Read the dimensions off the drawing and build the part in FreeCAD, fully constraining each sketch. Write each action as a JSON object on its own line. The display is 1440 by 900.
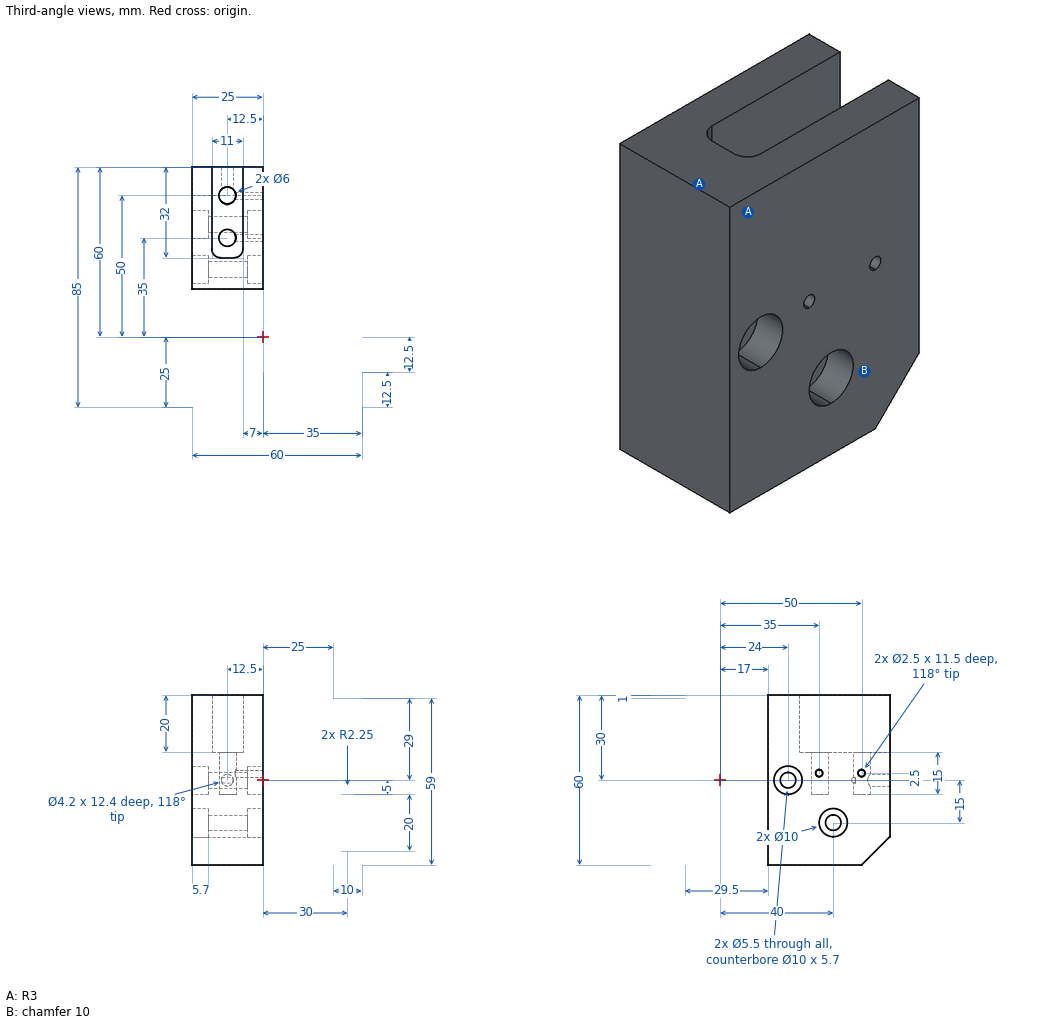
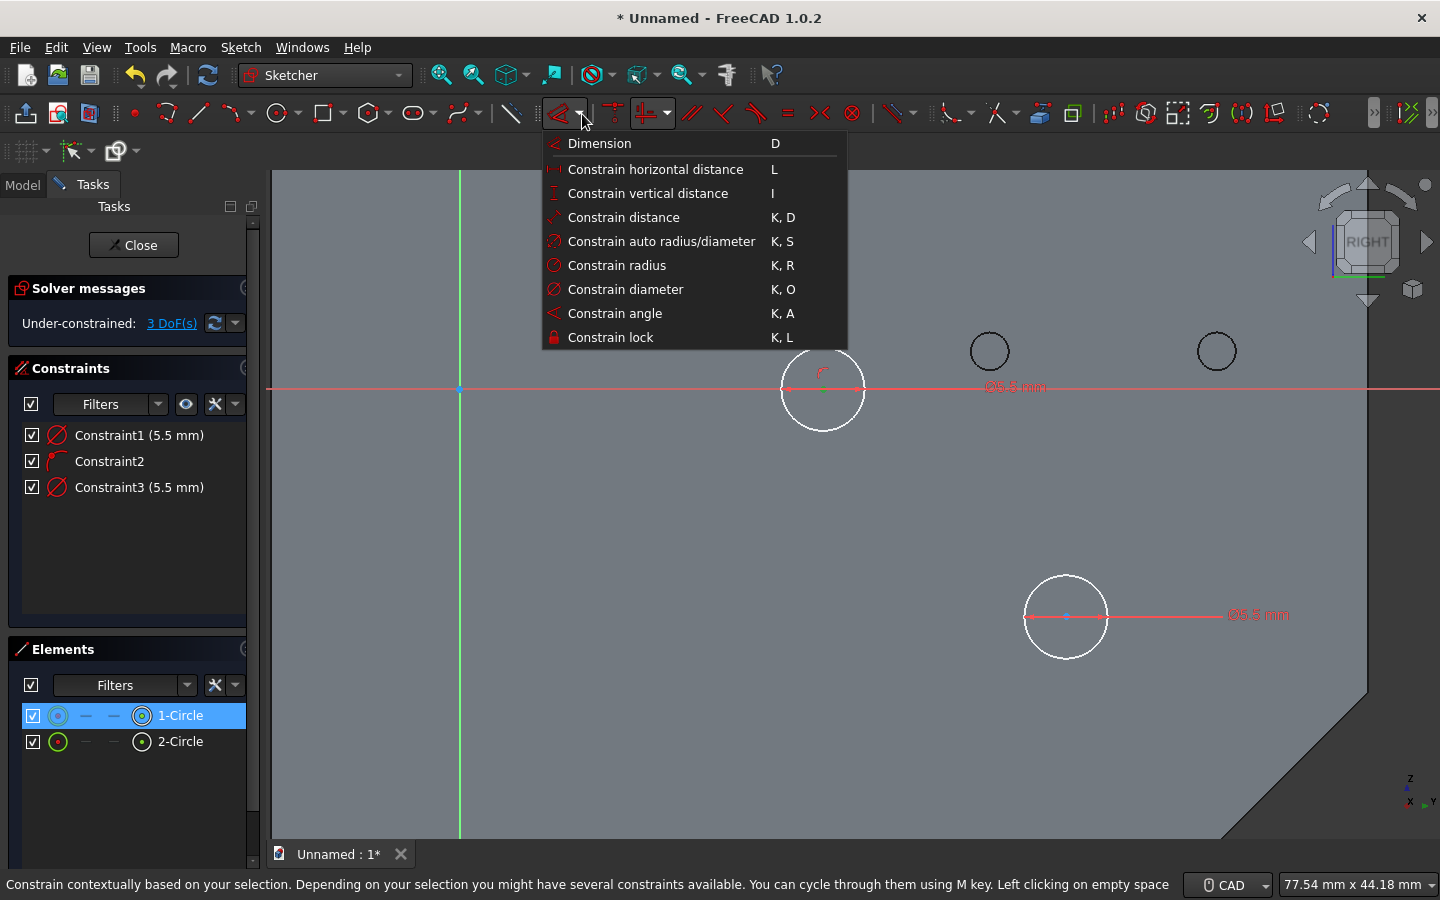
{"action": "left_click", "coordinate": [695, 169]}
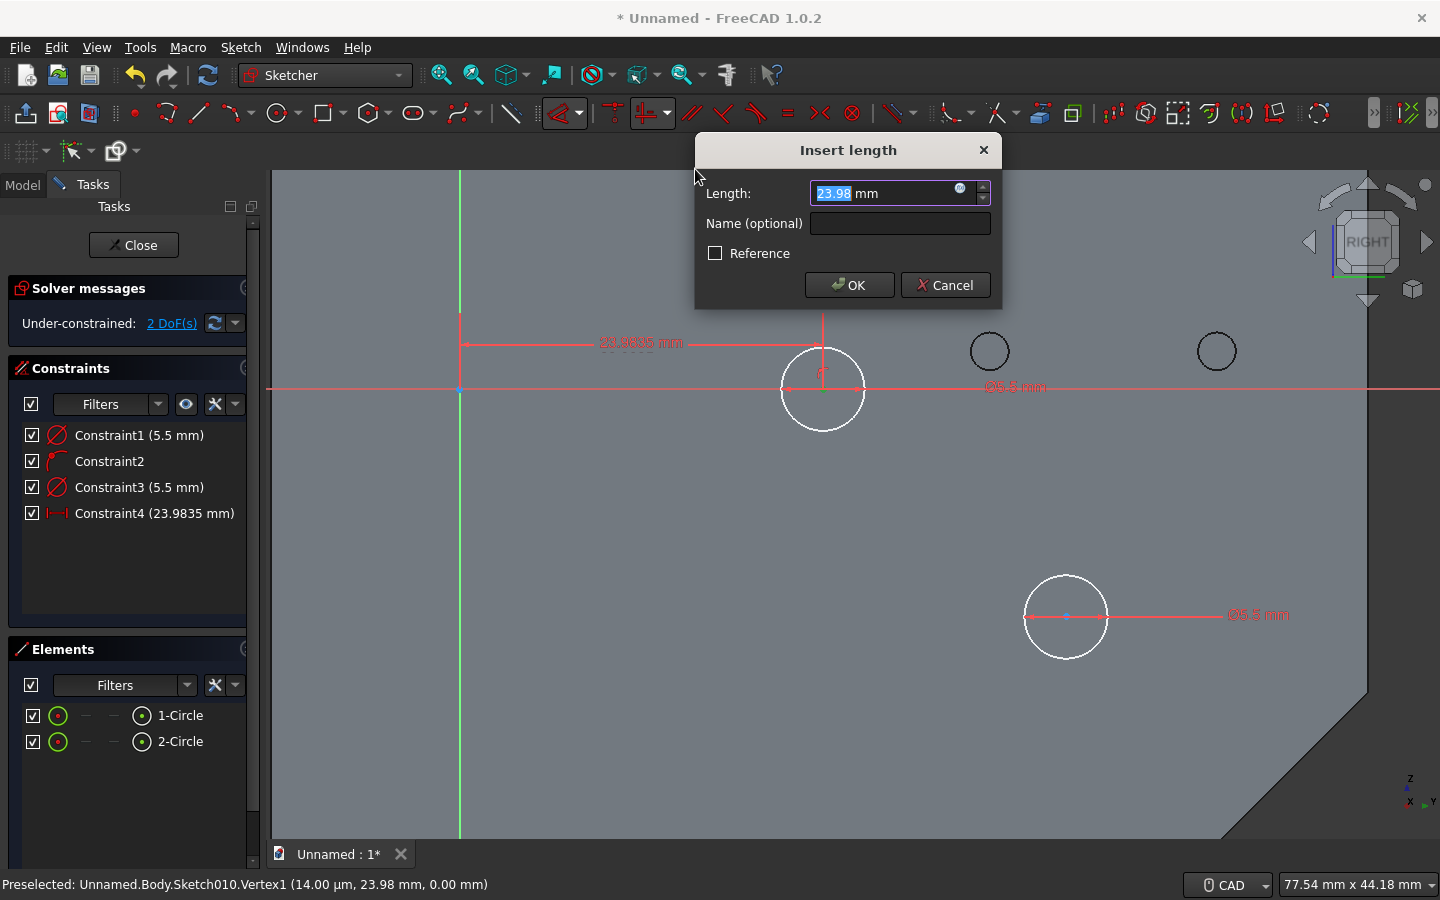
{"action": "type", "text": "24"}
{"action": "key", "text": "Return"}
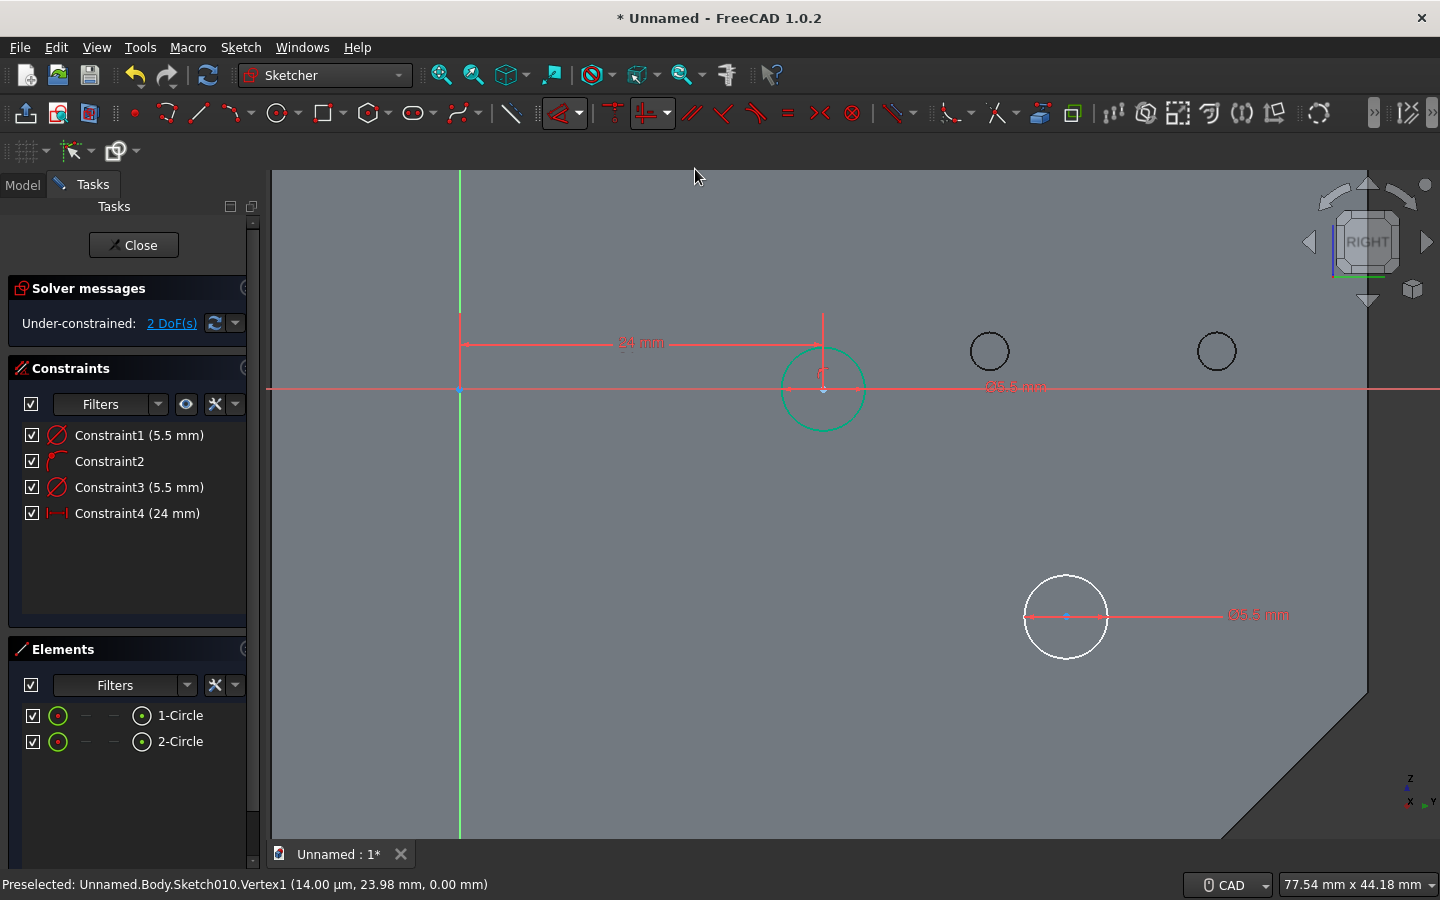
{"action": "left_click", "coordinate": [1066, 617]}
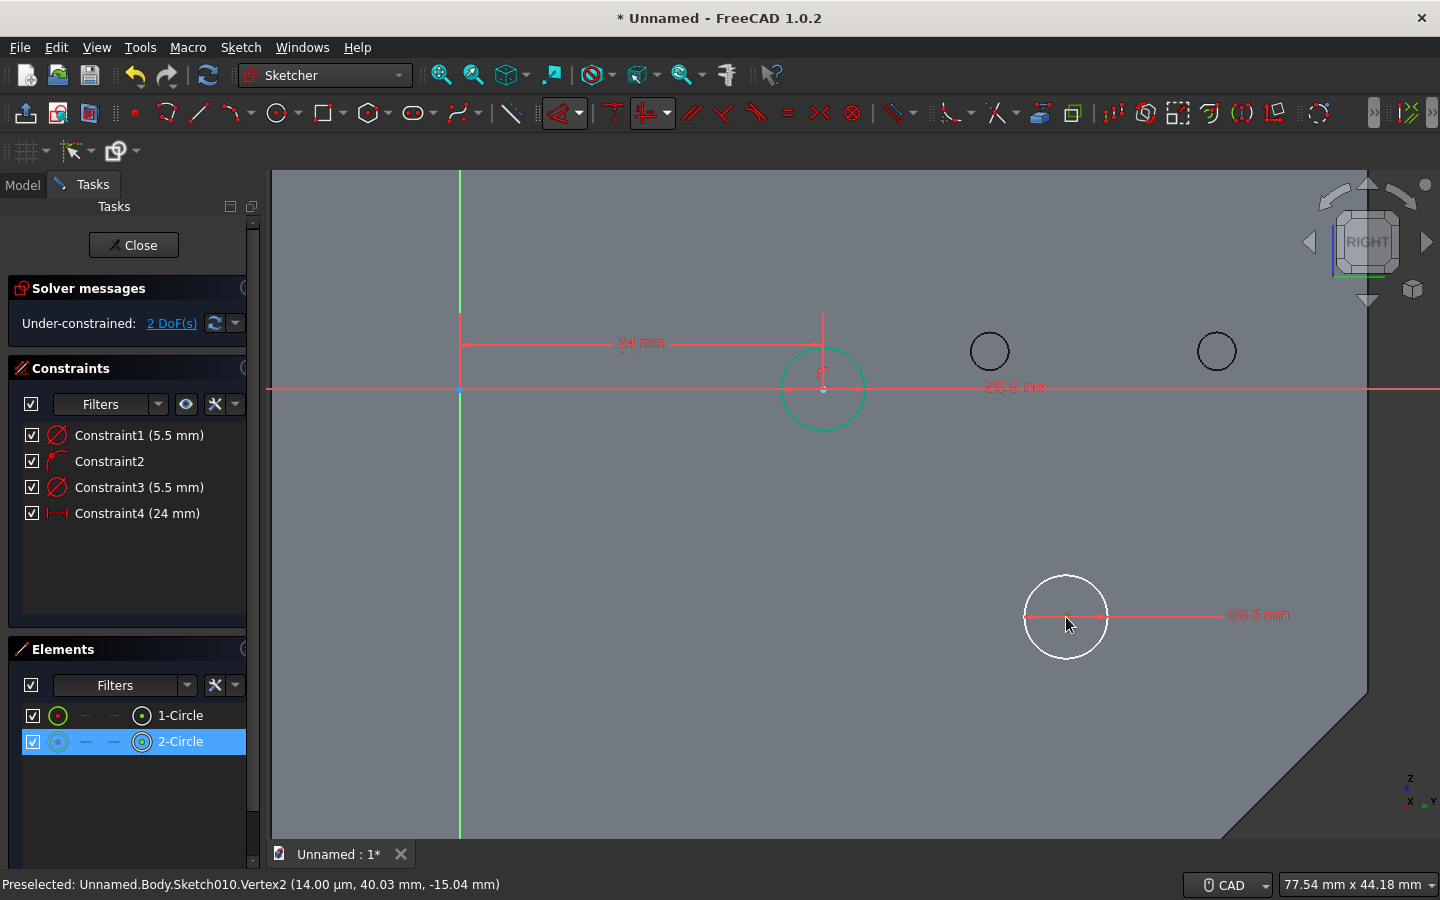
{"action": "key", "text": "l"}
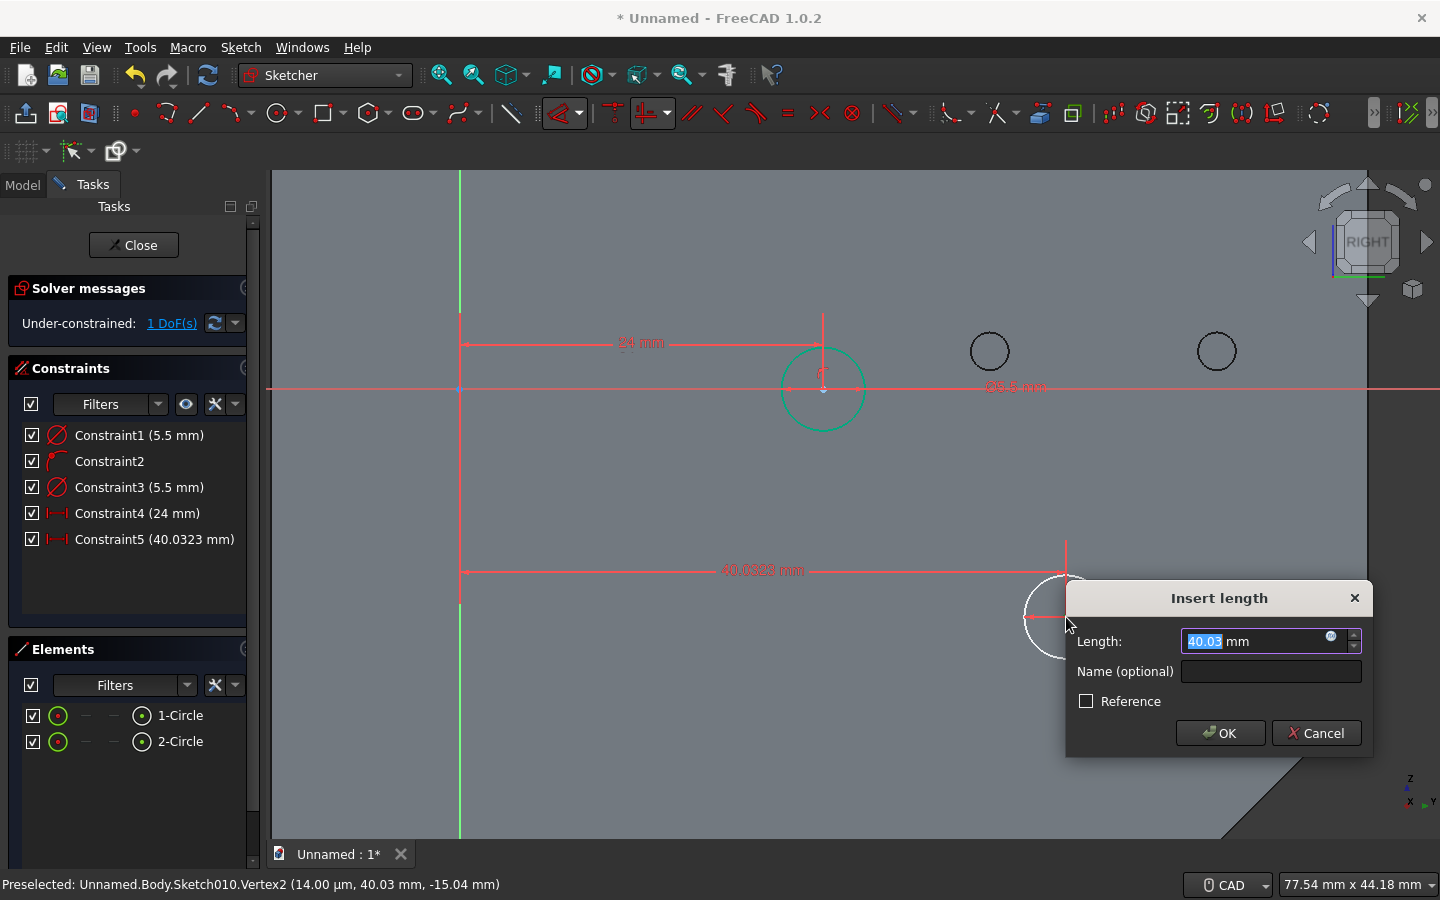
{"action": "type", "text": "40"}
{"action": "key", "text": "Return"}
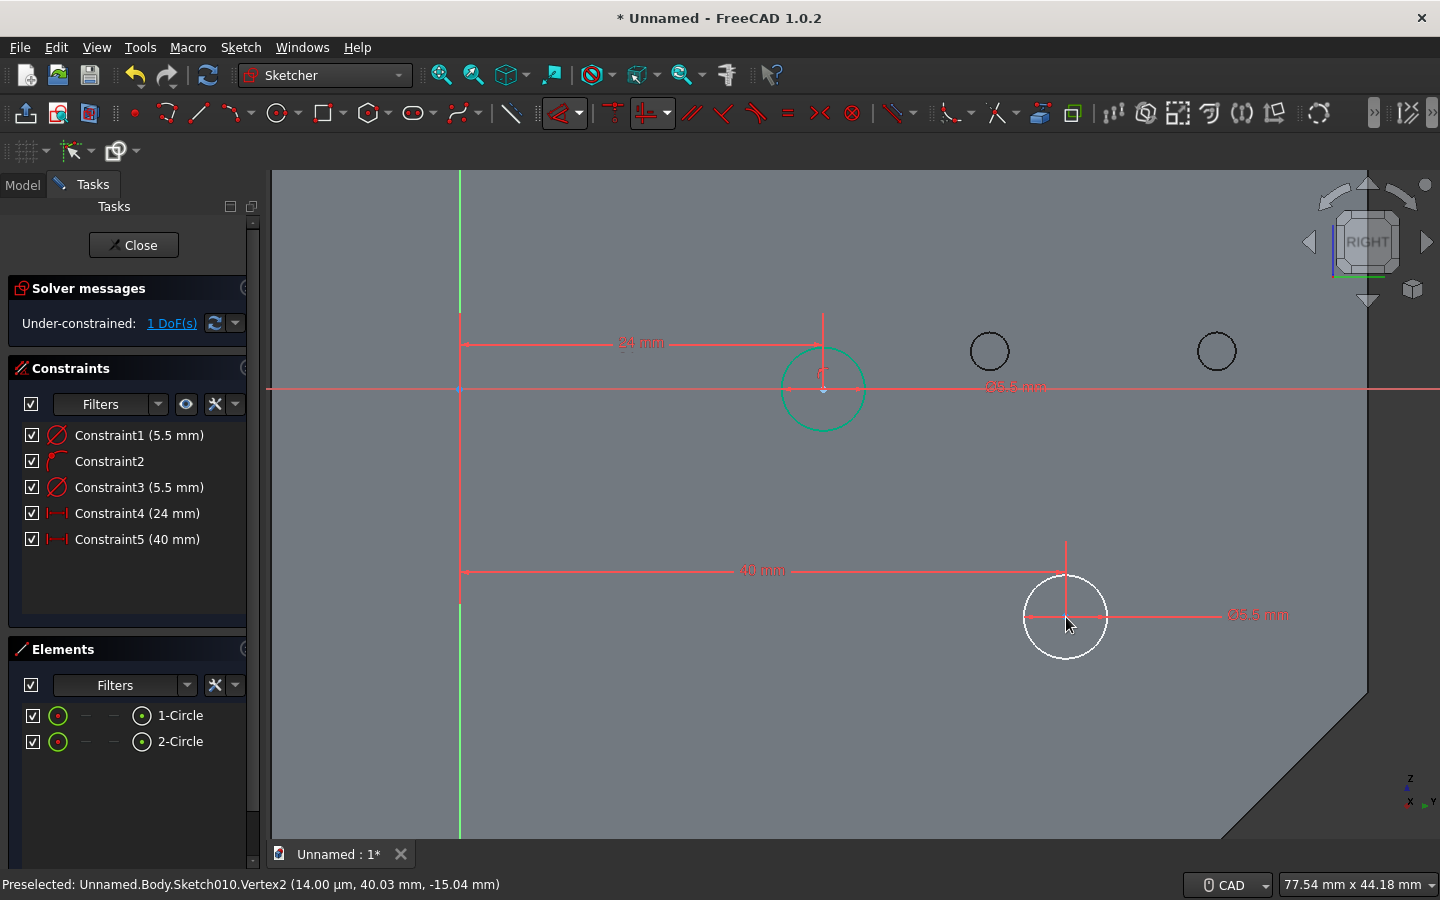
{"action": "left_click", "coordinate": [1066, 617]}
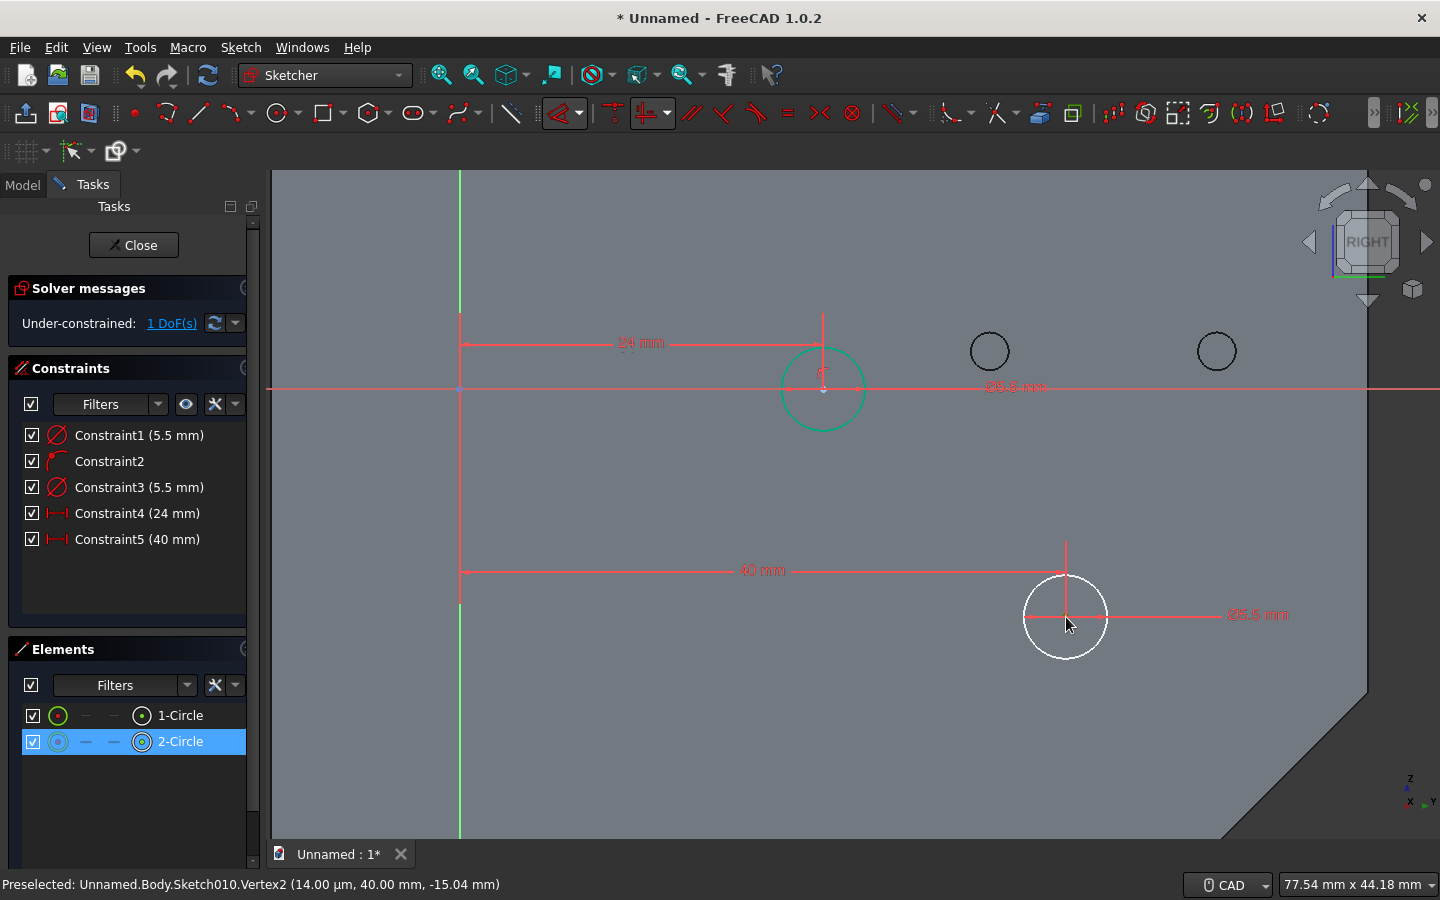
{"action": "left_click", "coordinate": [582, 114]}